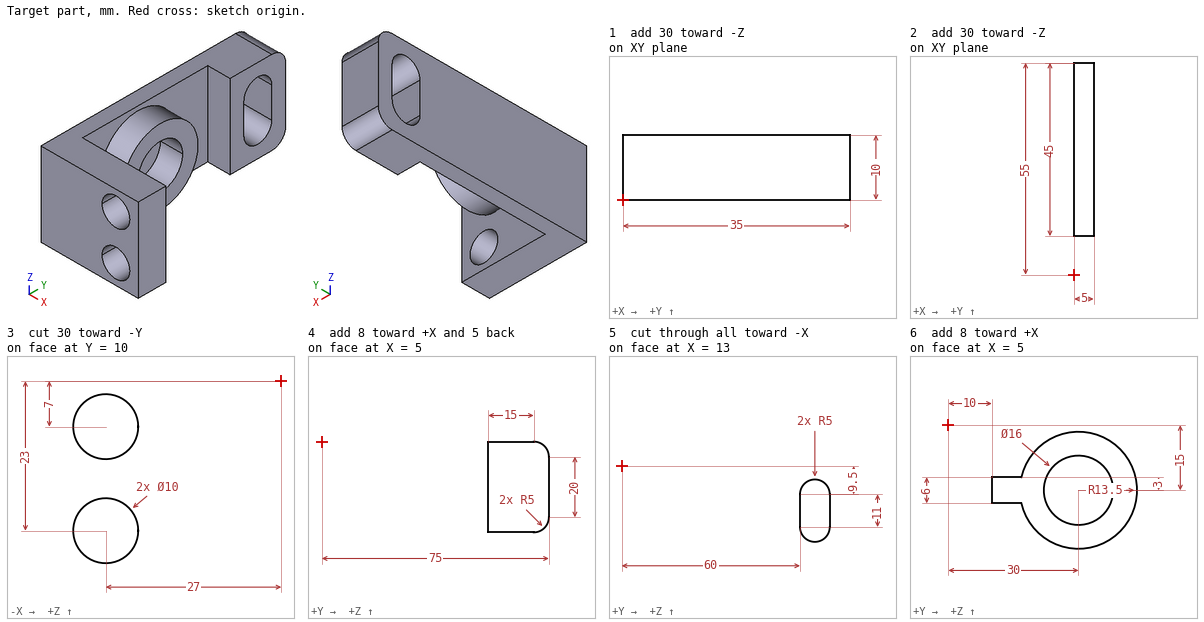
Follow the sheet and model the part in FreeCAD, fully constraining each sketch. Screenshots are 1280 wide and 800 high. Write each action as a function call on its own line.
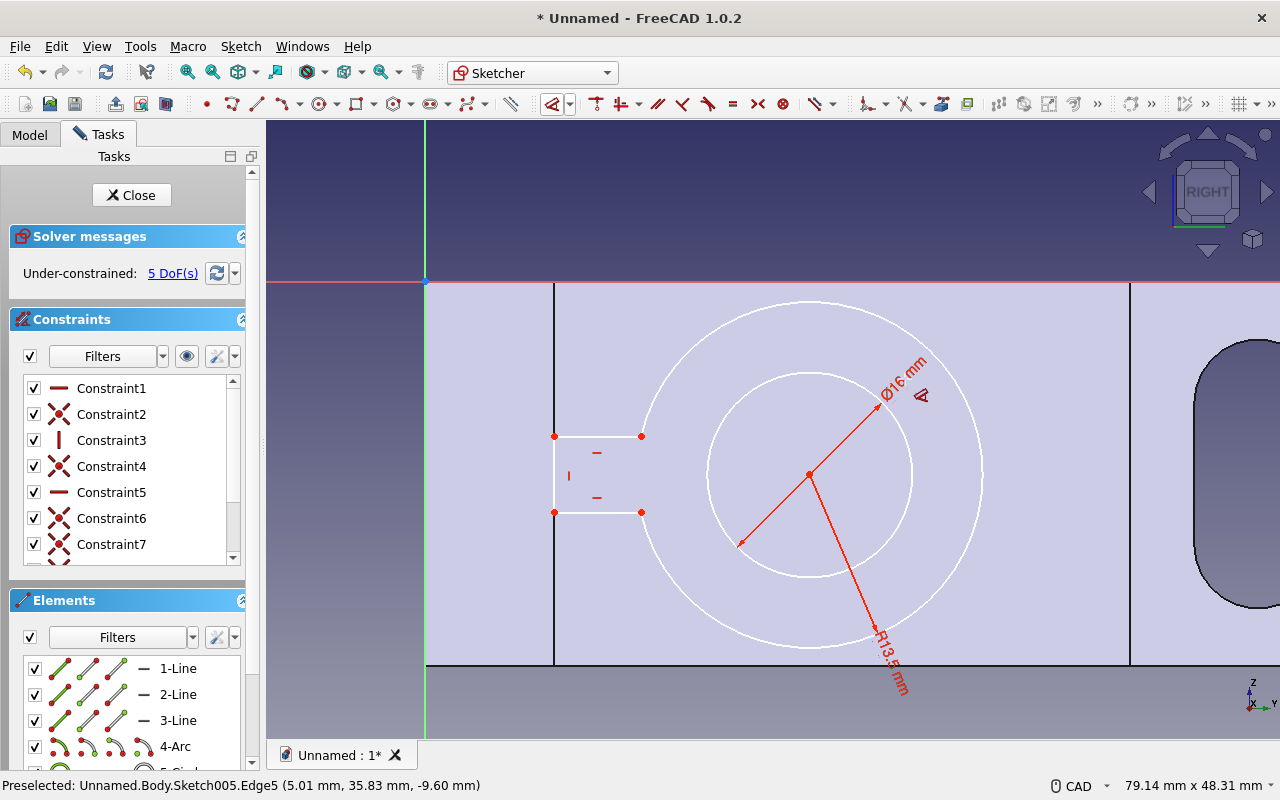
click(554, 460)
click(520, 475)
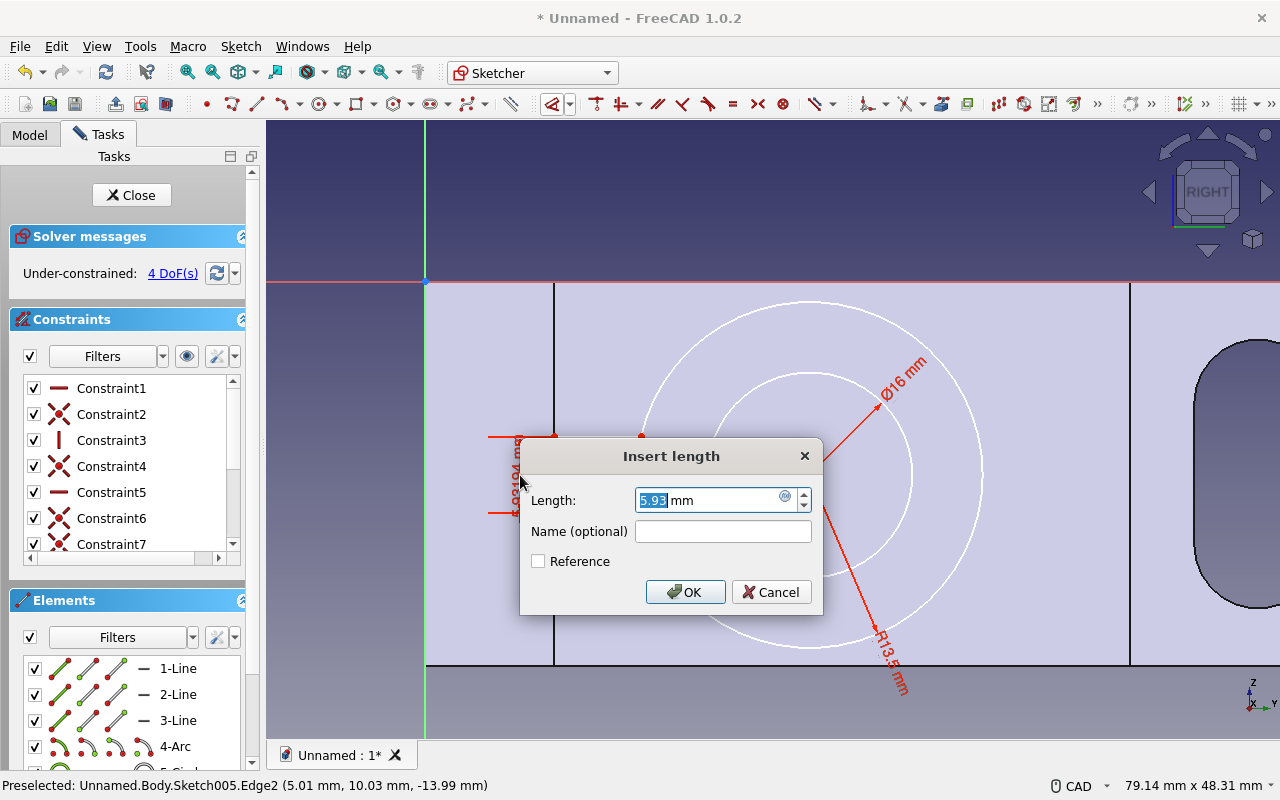
text(6)
key(Return)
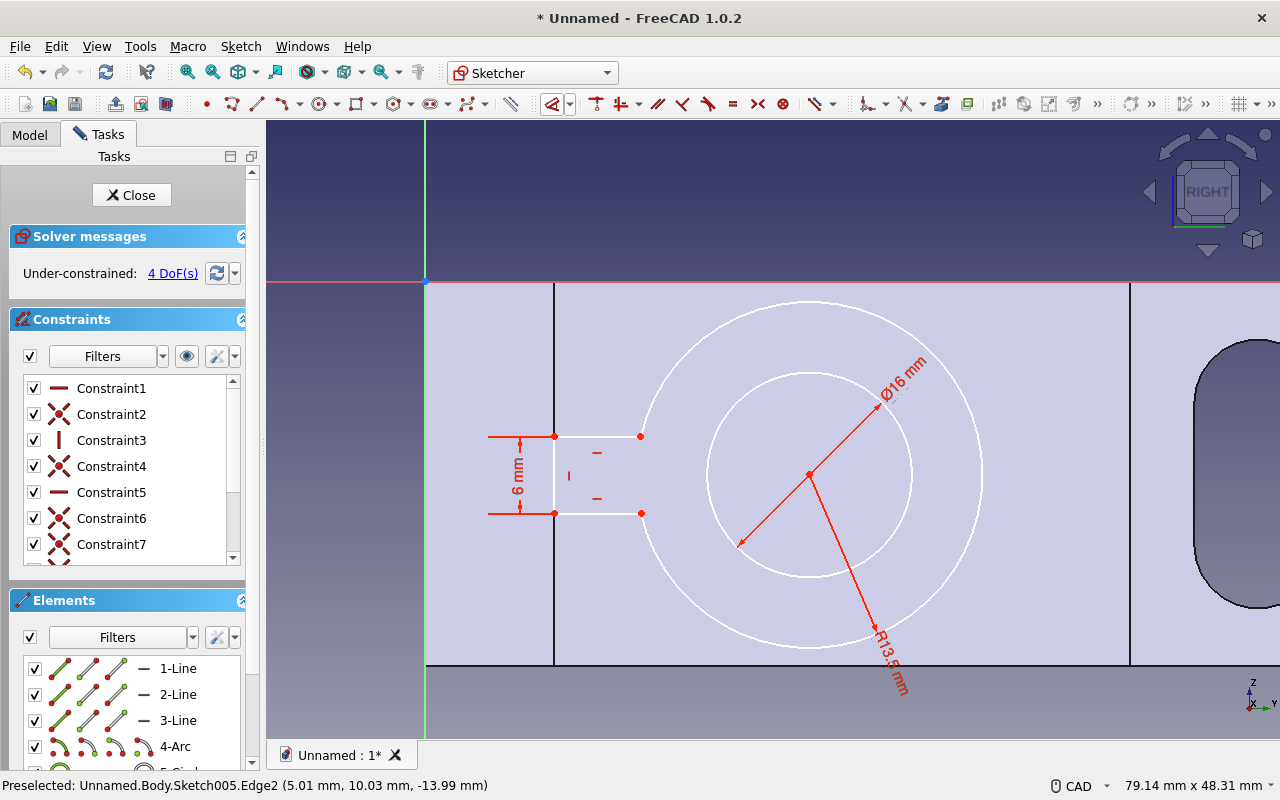
click(810, 475)
click(617, 248)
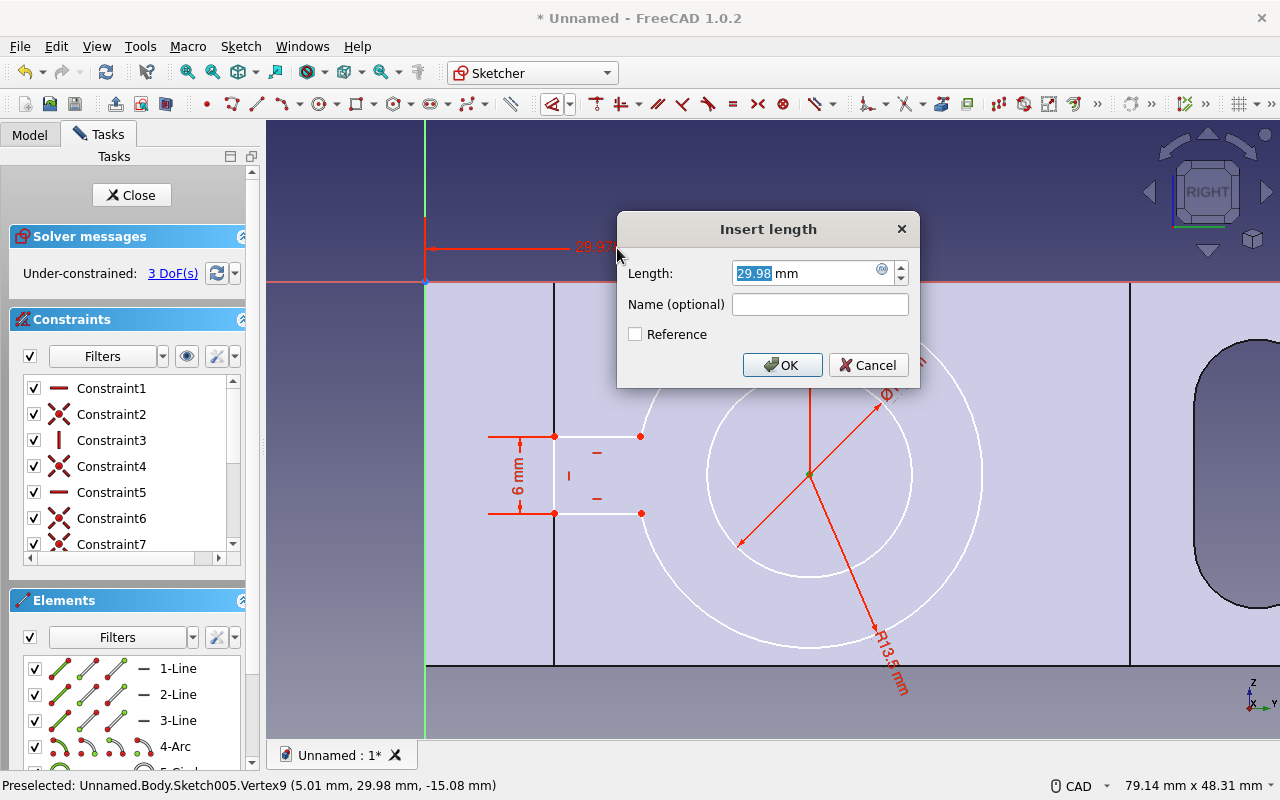
text(30)
key(Return)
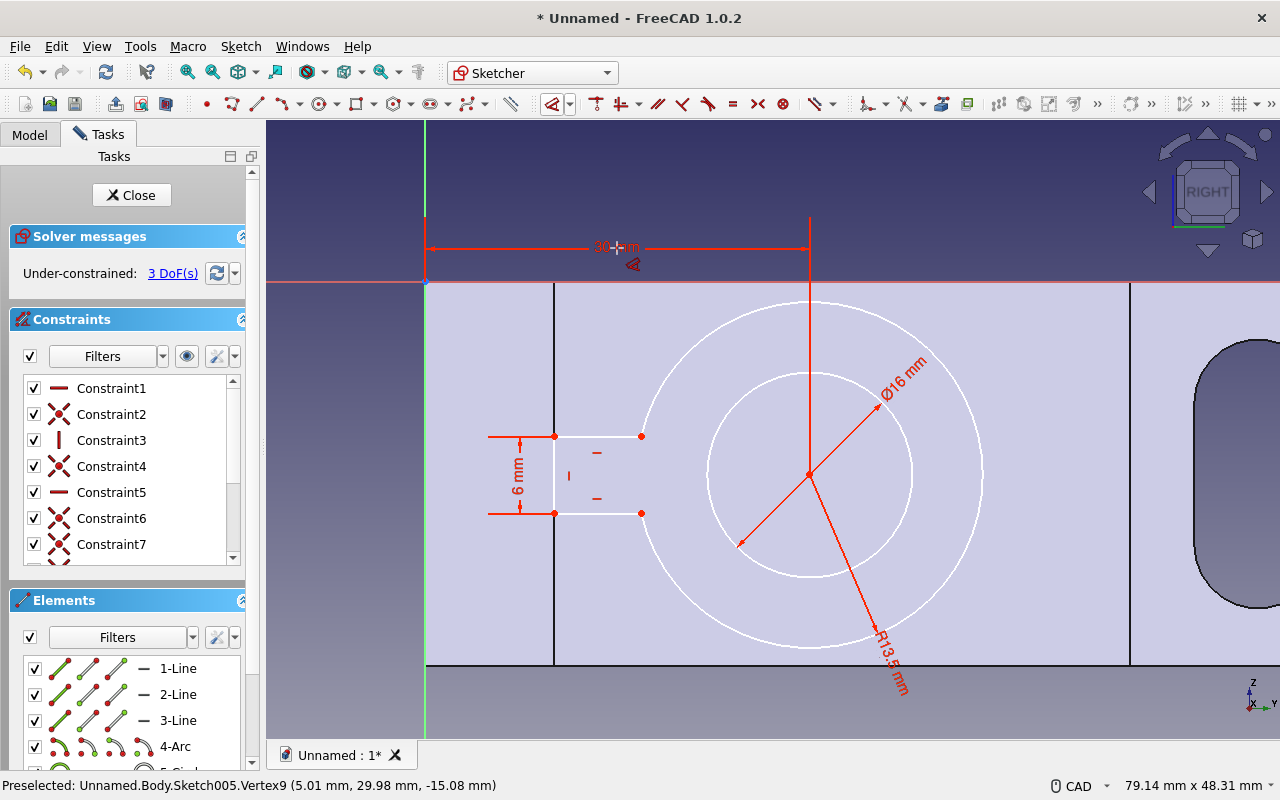
click(810, 475)
click(391, 378)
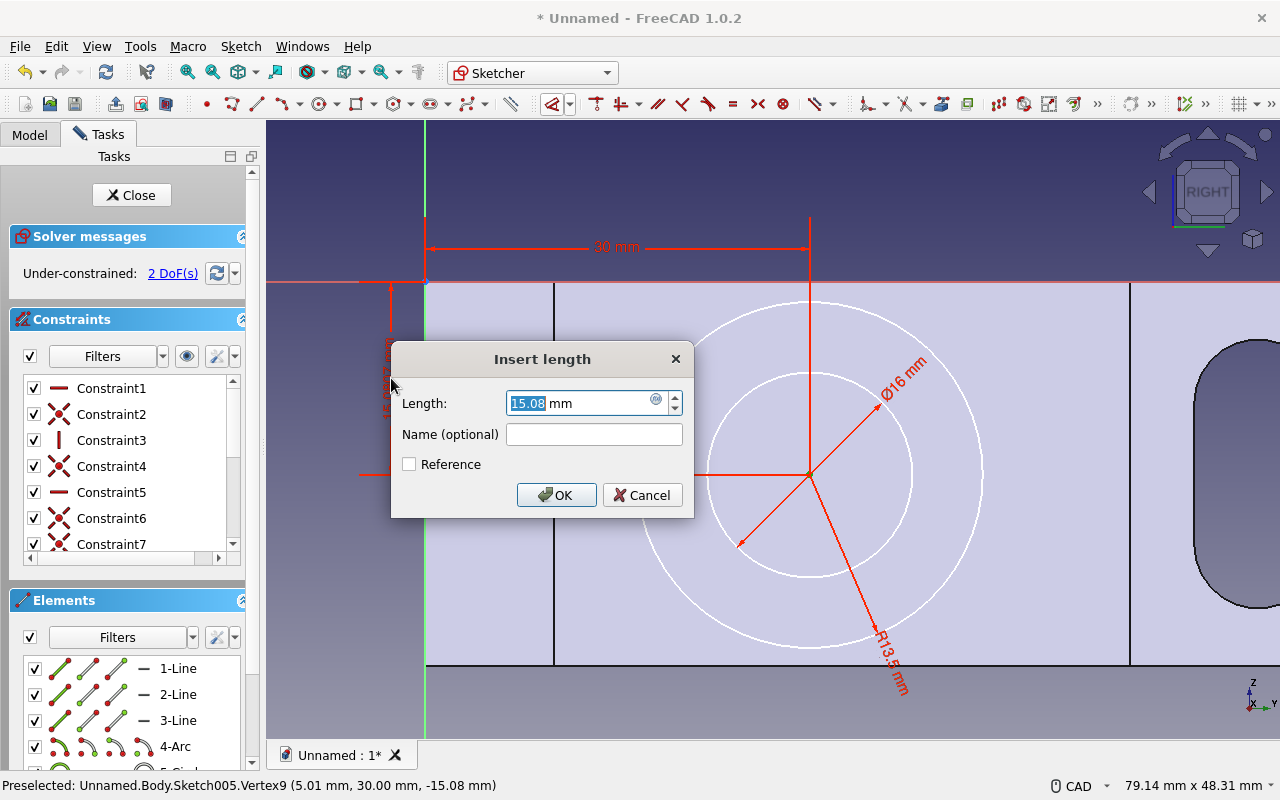
text(15)
key(Return)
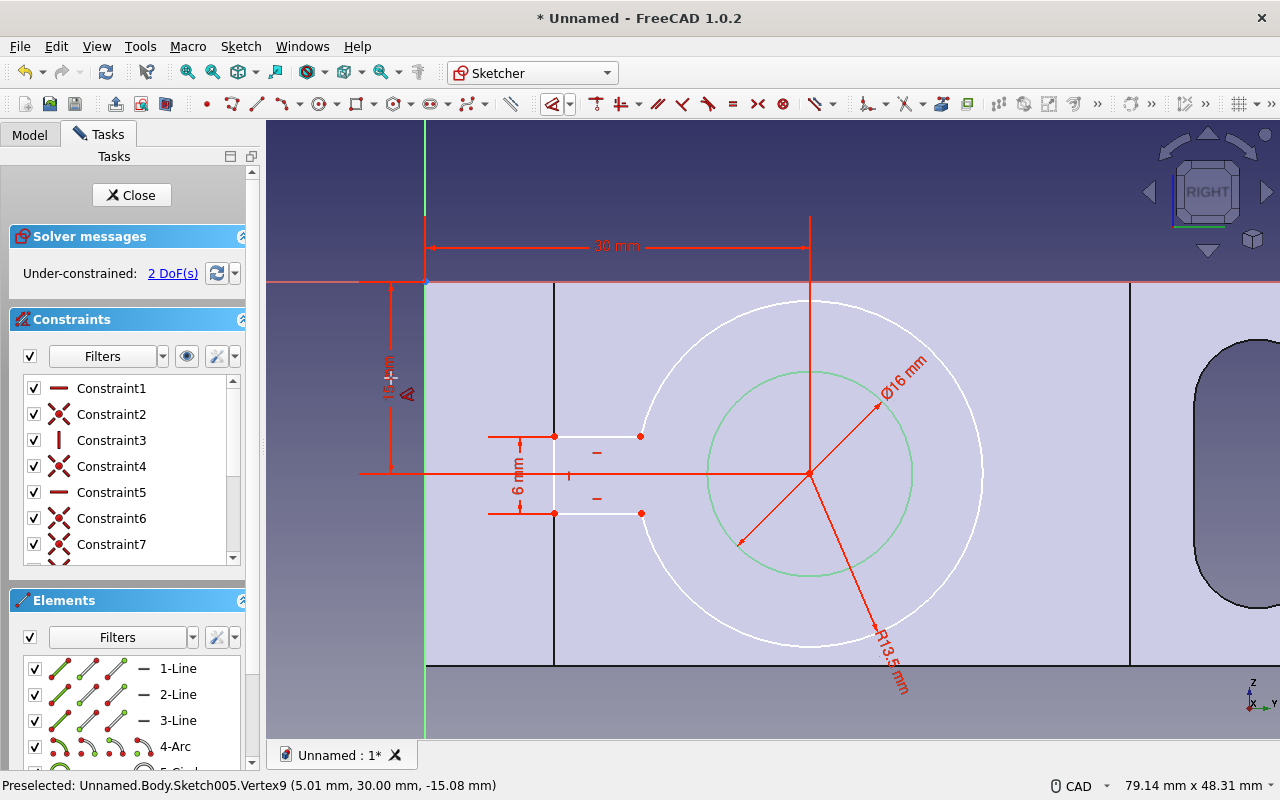
click(641, 437)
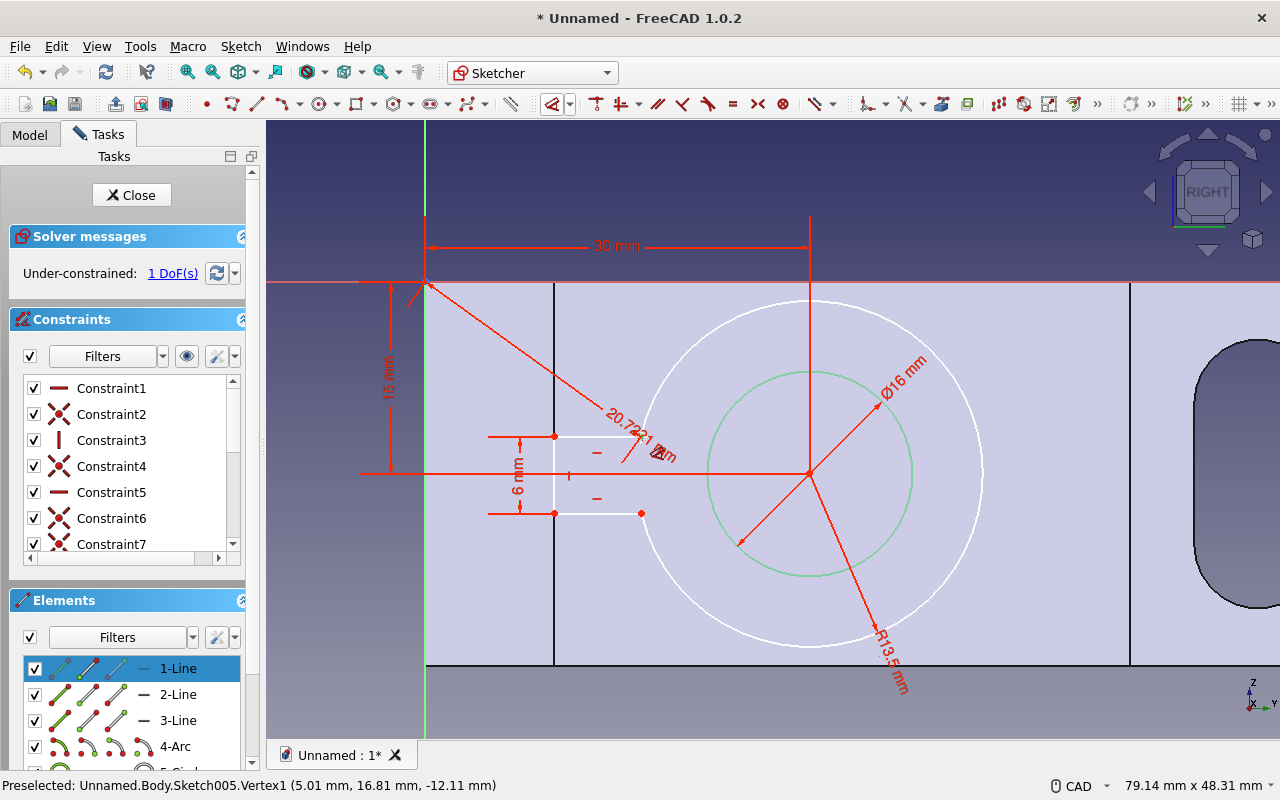
click(810, 474)
click(844, 455)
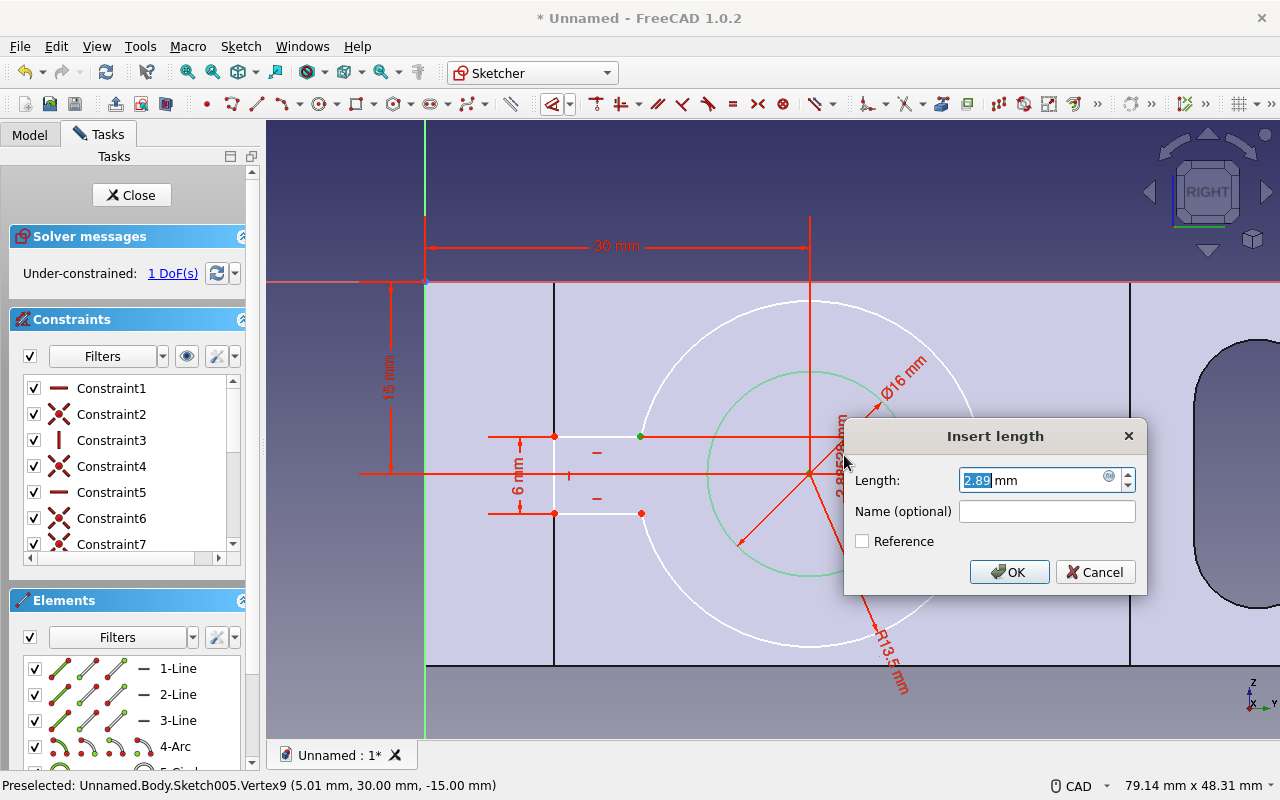
text(3)
key(Return)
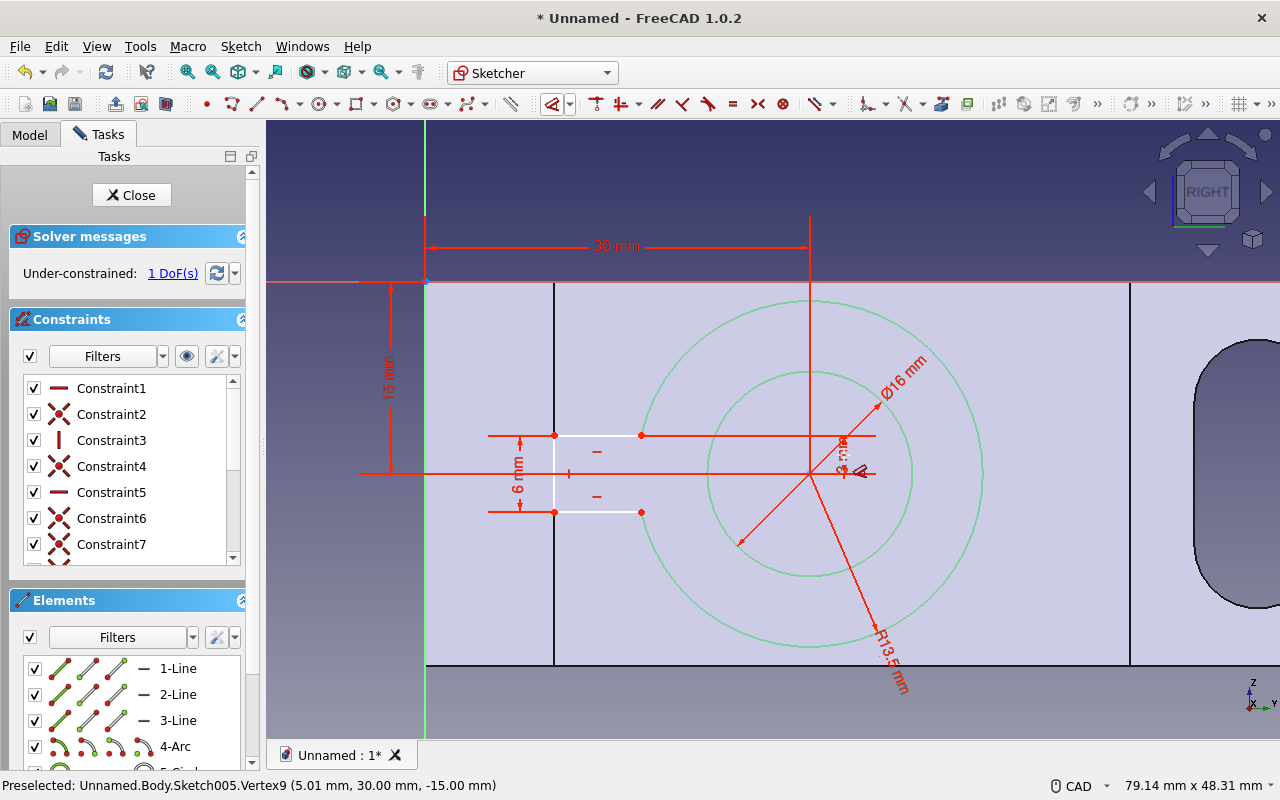
click(554, 436)
click(490, 248)